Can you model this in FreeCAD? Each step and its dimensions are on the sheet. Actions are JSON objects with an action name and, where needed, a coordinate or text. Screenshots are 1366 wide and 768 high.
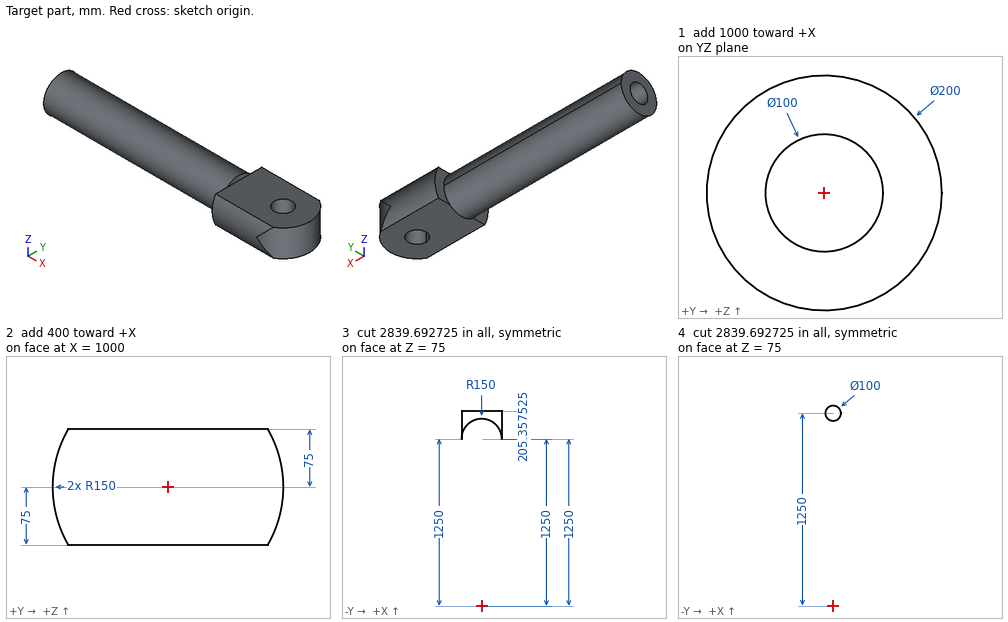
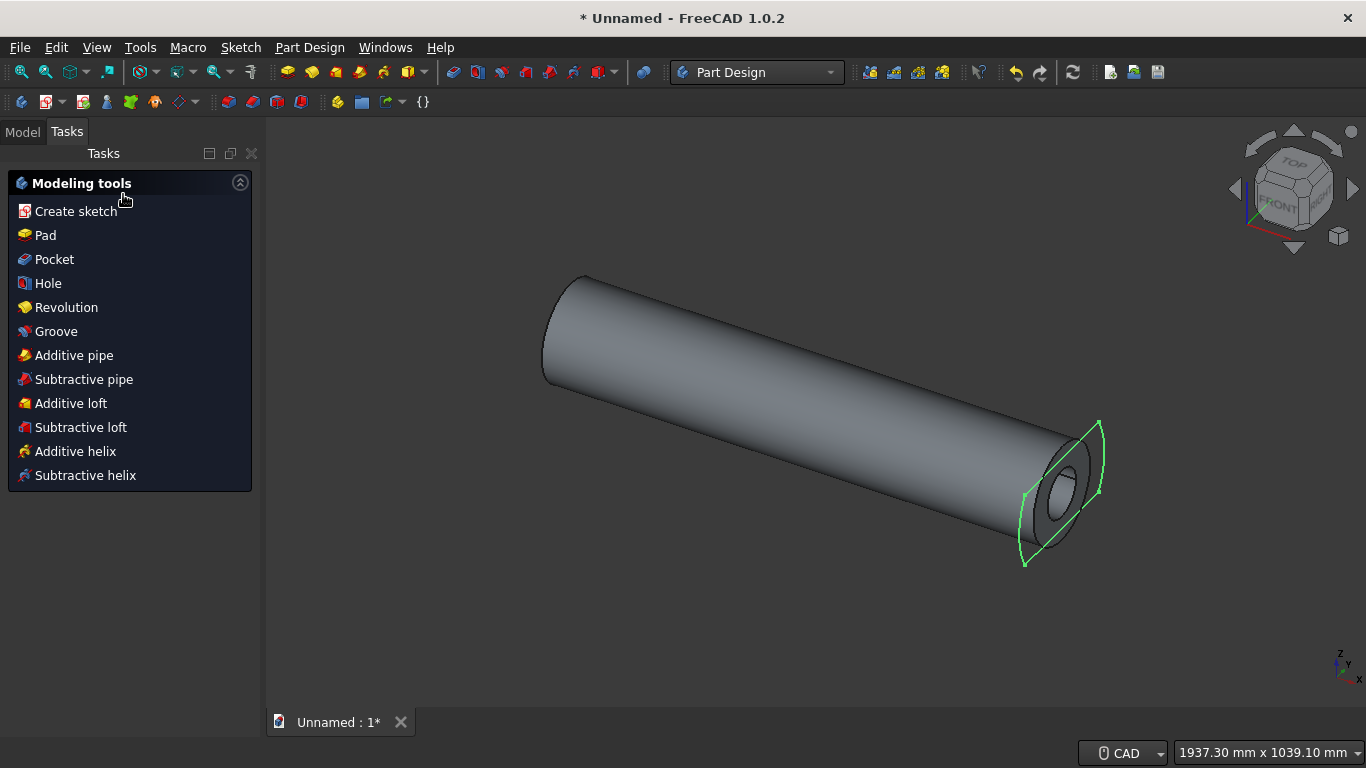
{"action": "left_click", "coordinate": [288, 72]}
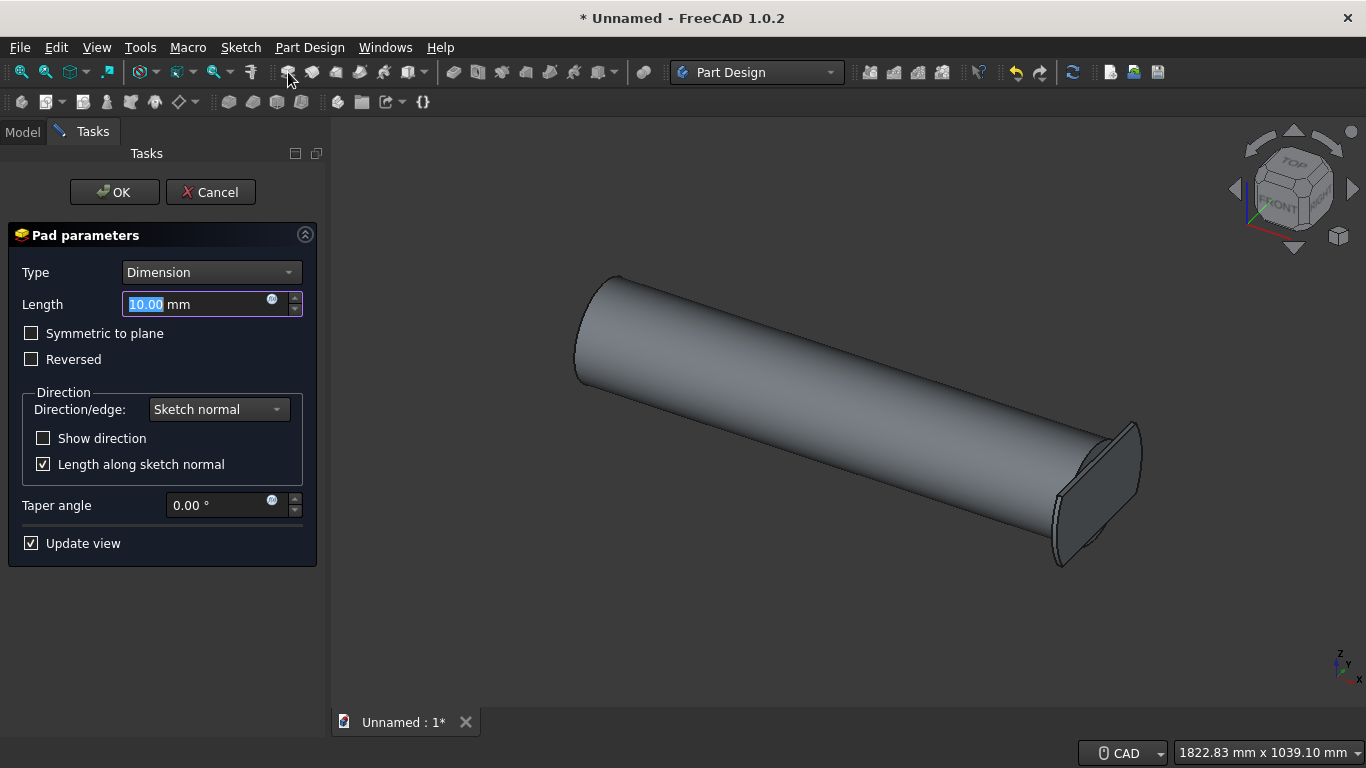
{"action": "type", "text": "400"}
{"action": "key", "text": "Tab"}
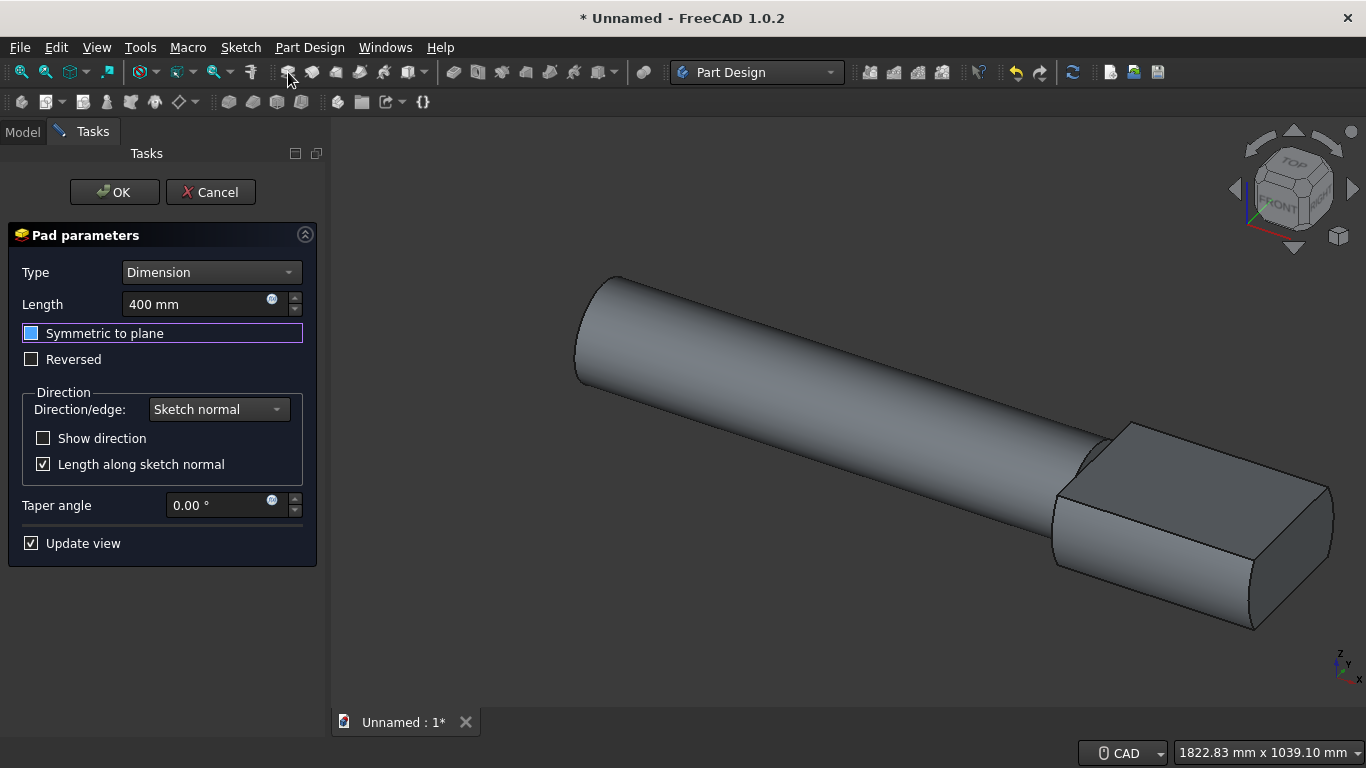
{"action": "left_click", "coordinate": [115, 192]}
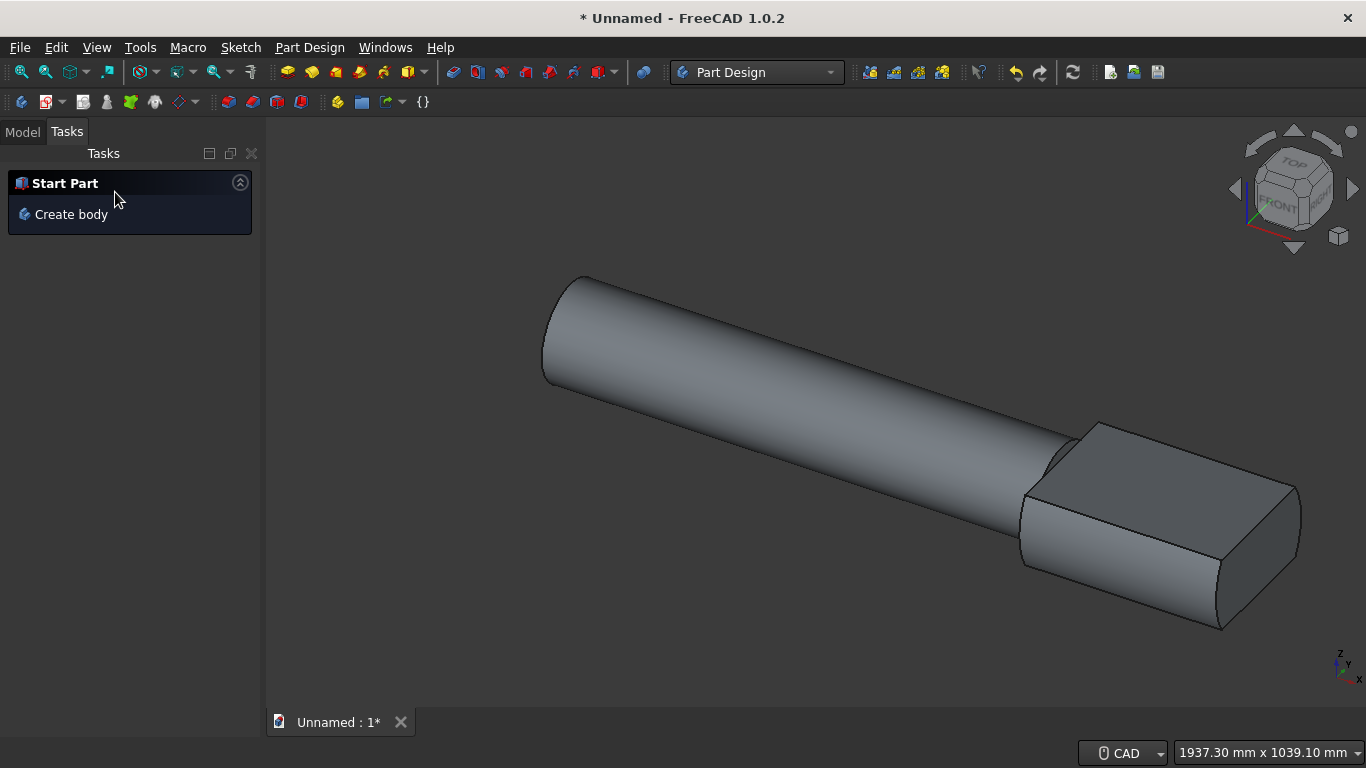
{"action": "left_click", "coordinate": [1188, 500]}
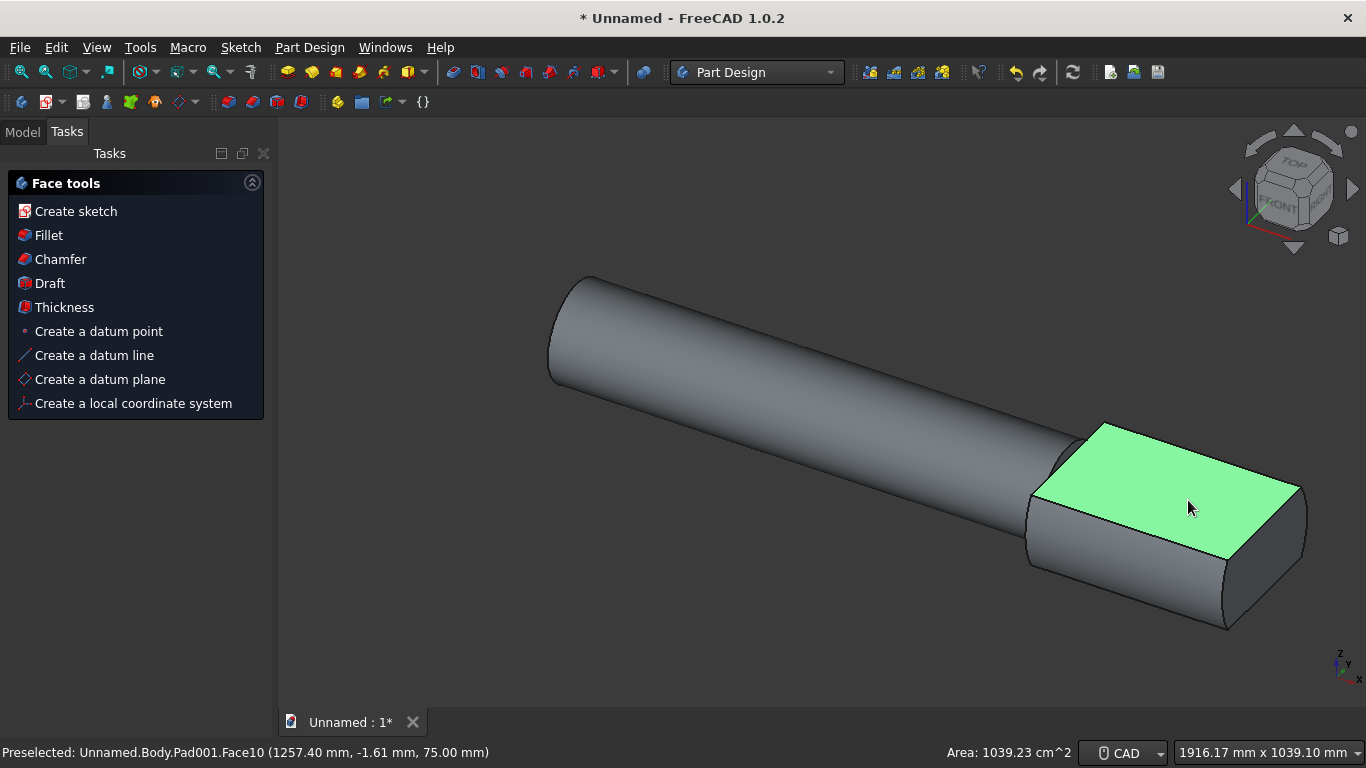
{"action": "left_click", "coordinate": [46, 102]}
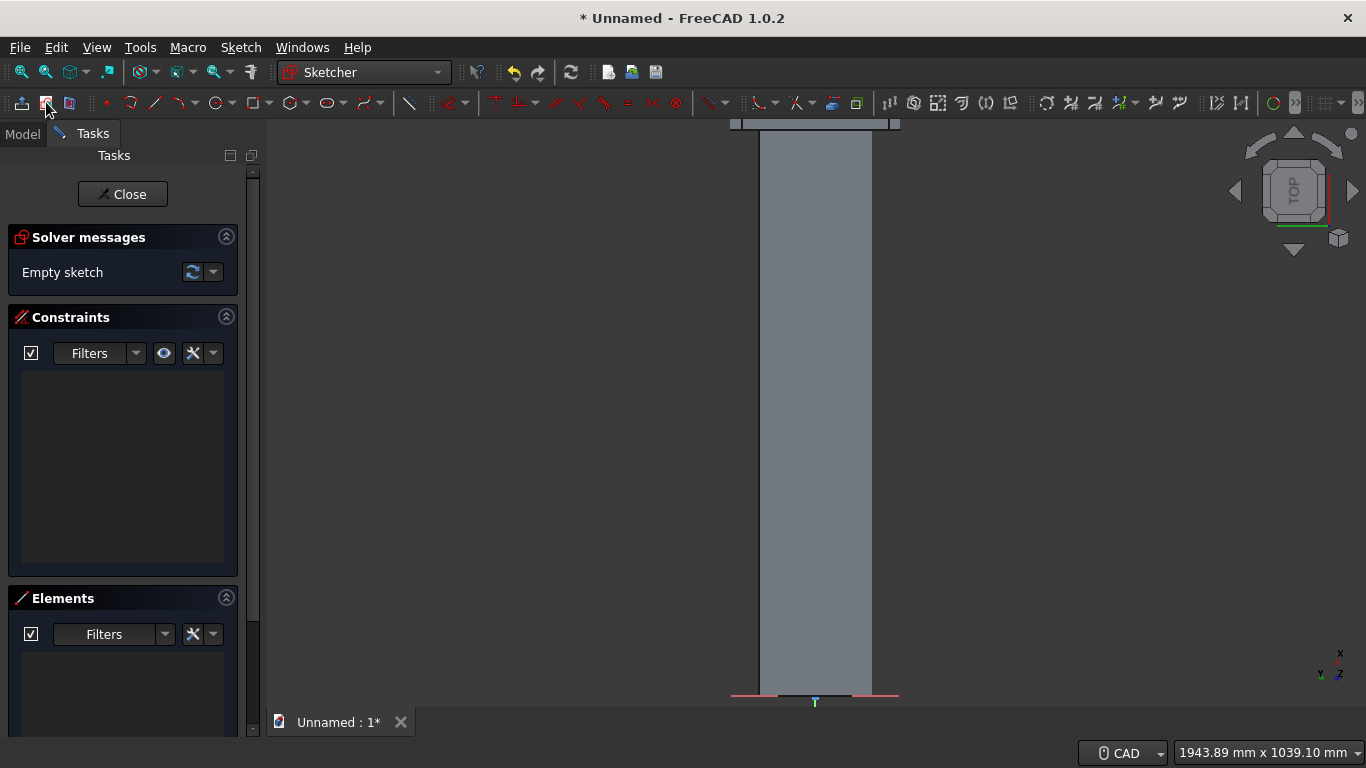
{"action": "left_click", "coordinate": [70, 104]}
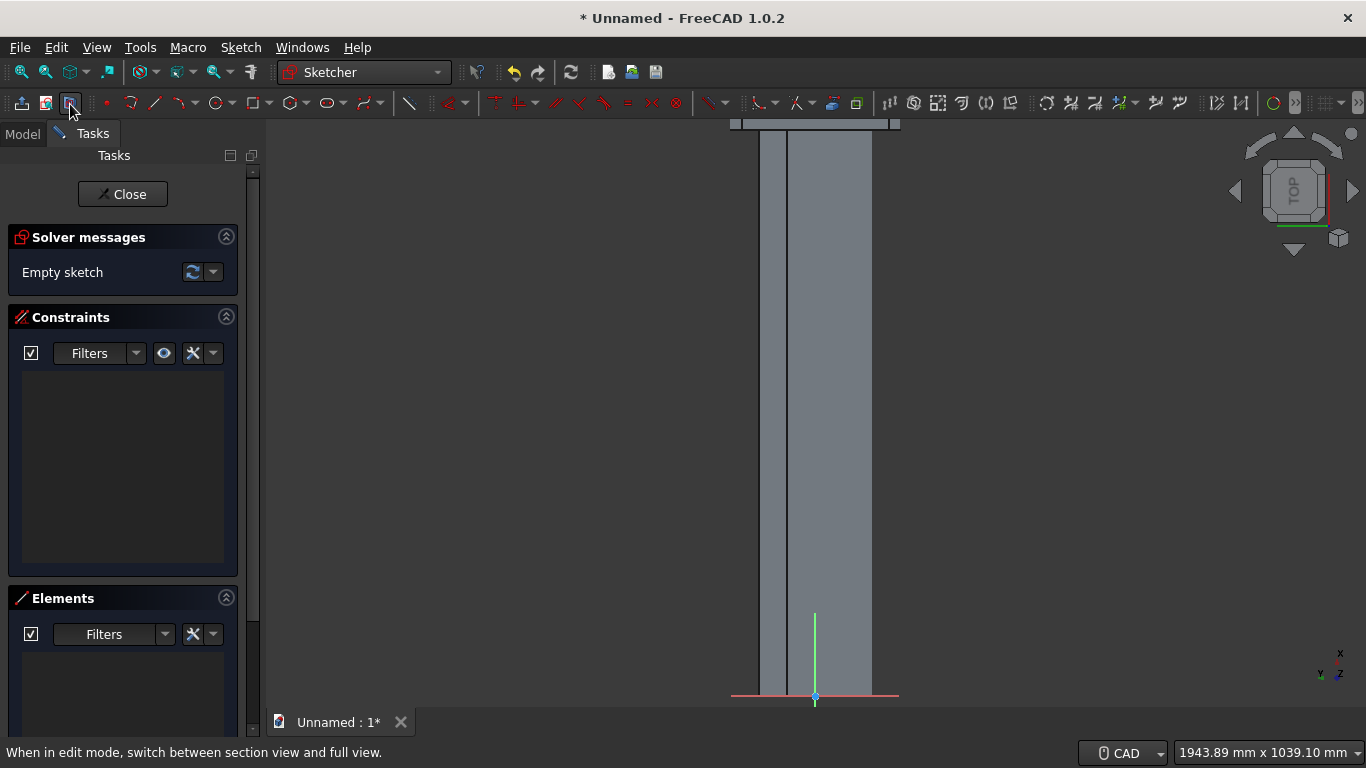
{"action": "scroll", "coordinate": [748, 413], "scroll_direction": "down", "scroll_amount": 5}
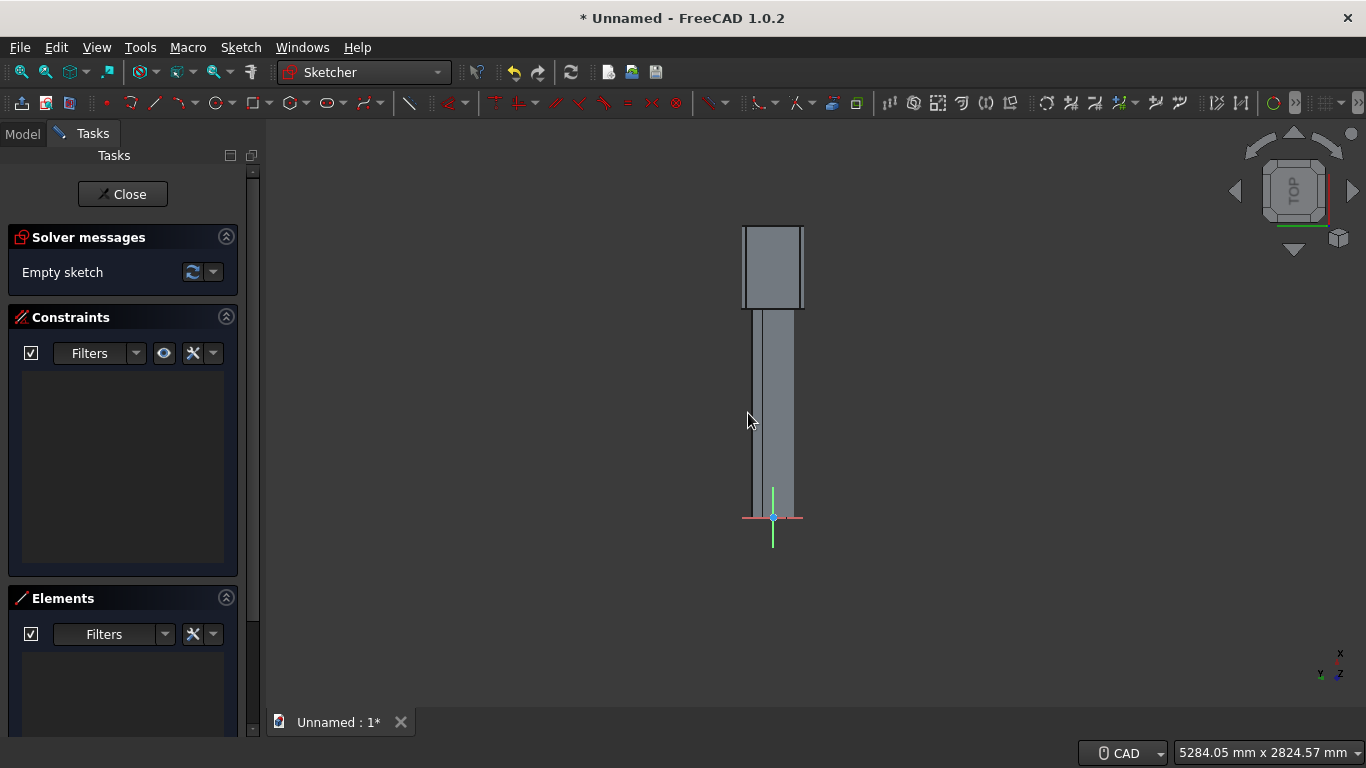
{"action": "scroll", "coordinate": [776, 214], "scroll_direction": "up", "scroll_amount": 11}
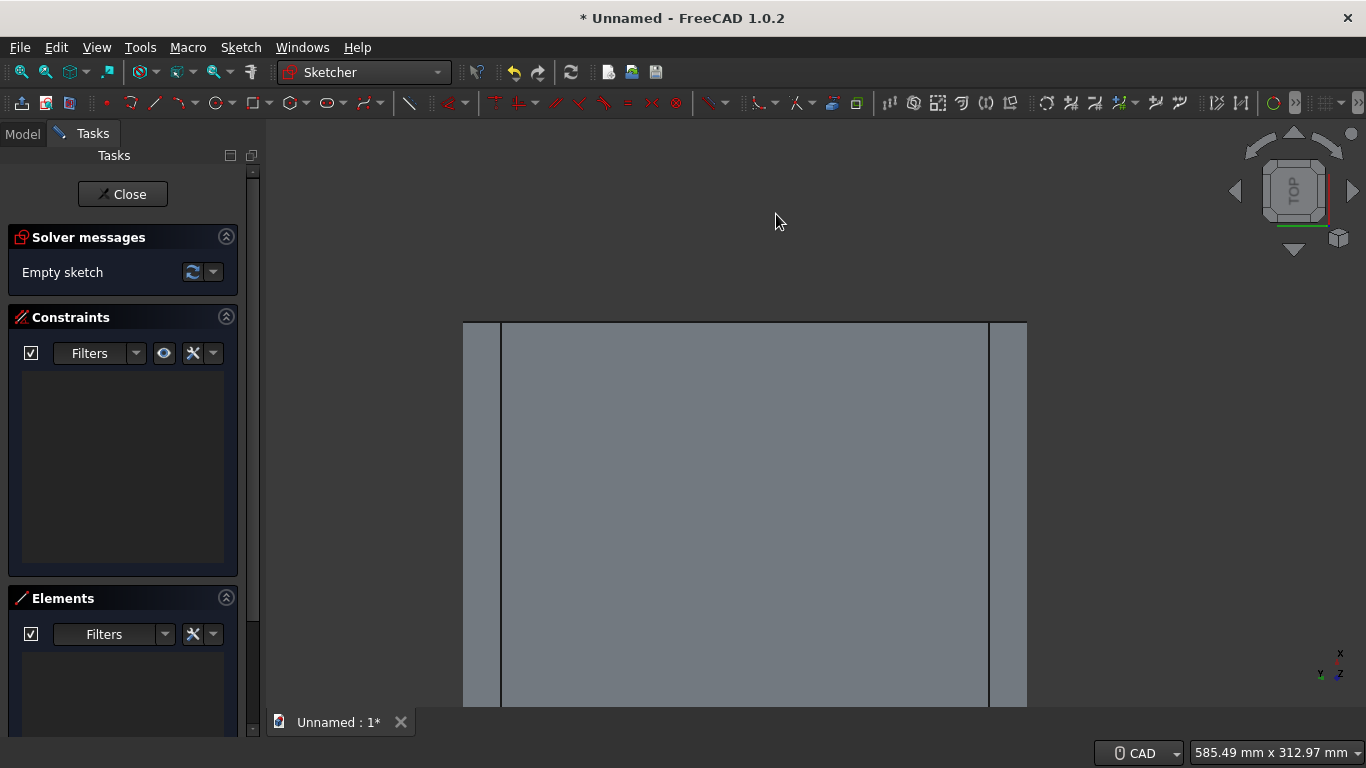
{"action": "left_click", "coordinate": [132, 104]}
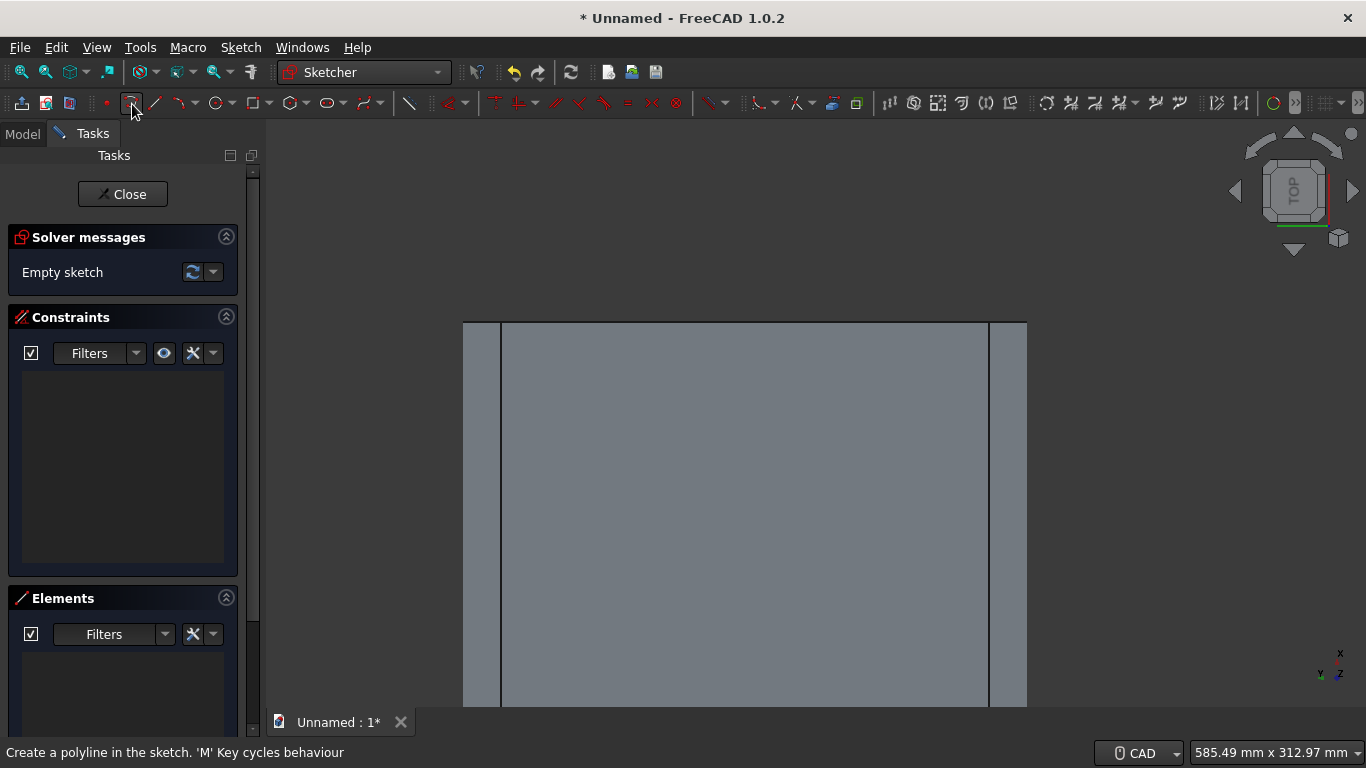
{"action": "left_click", "coordinate": [1027, 604]}
{"action": "left_click", "coordinate": [1027, 218]}
{"action": "left_click", "coordinate": [463, 218]}
{"action": "left_click", "coordinate": [463, 604]}
{"action": "right_click", "coordinate": [463, 604]}